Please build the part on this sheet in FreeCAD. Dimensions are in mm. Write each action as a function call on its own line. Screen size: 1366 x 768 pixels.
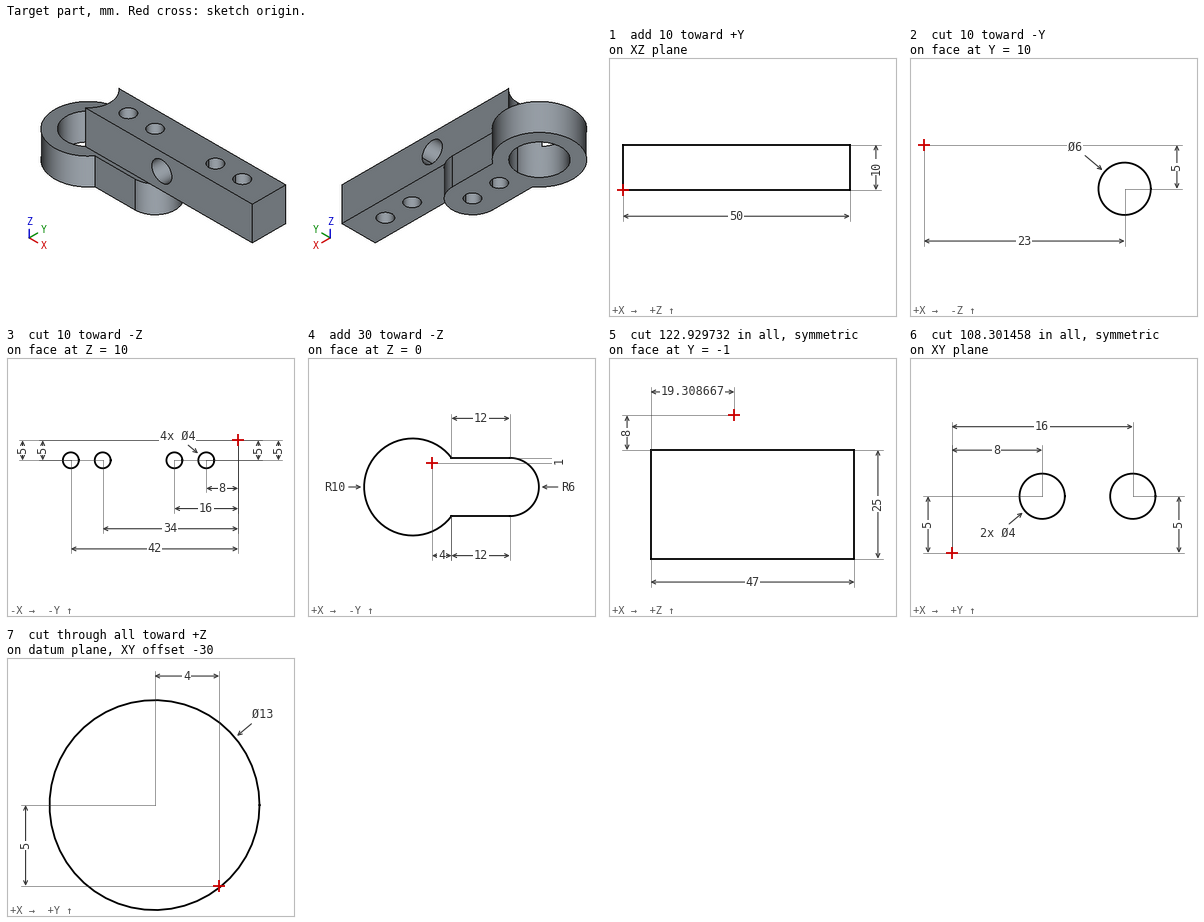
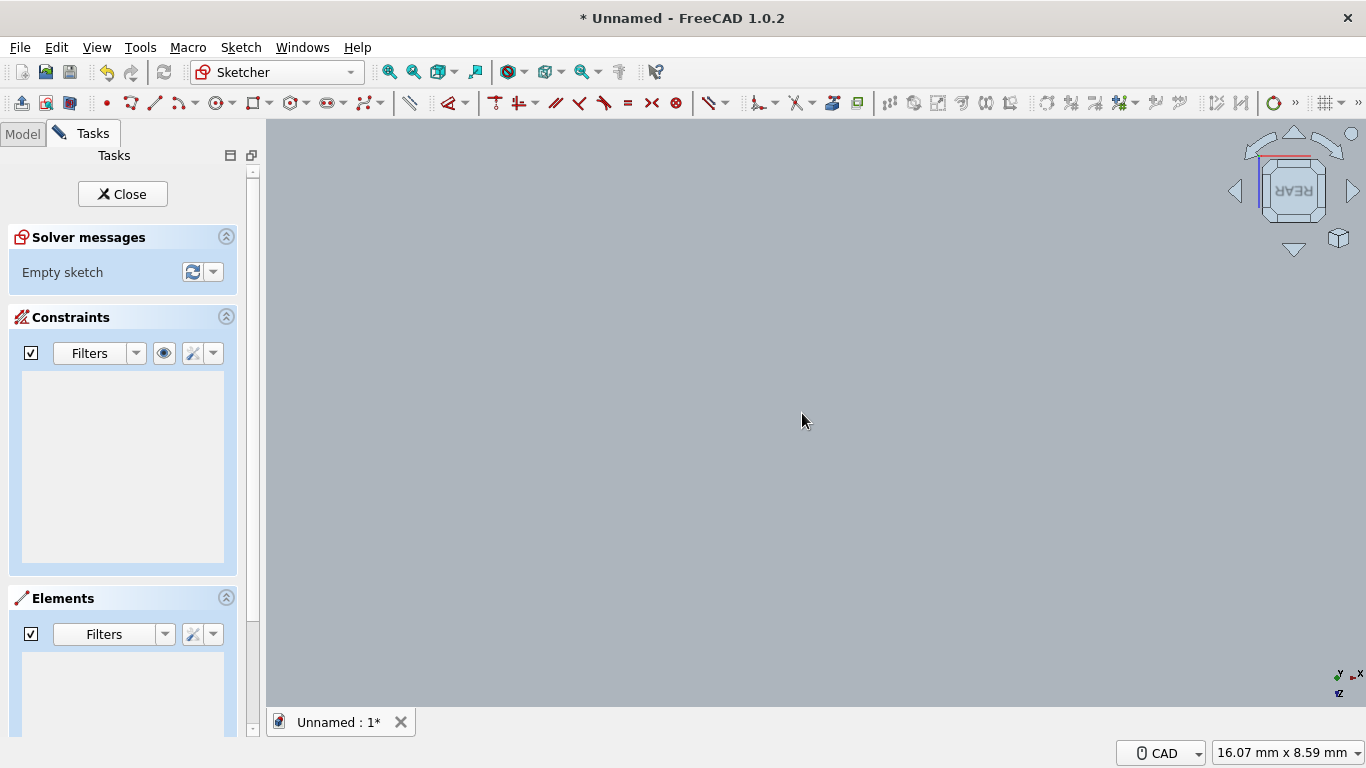
click(216, 104)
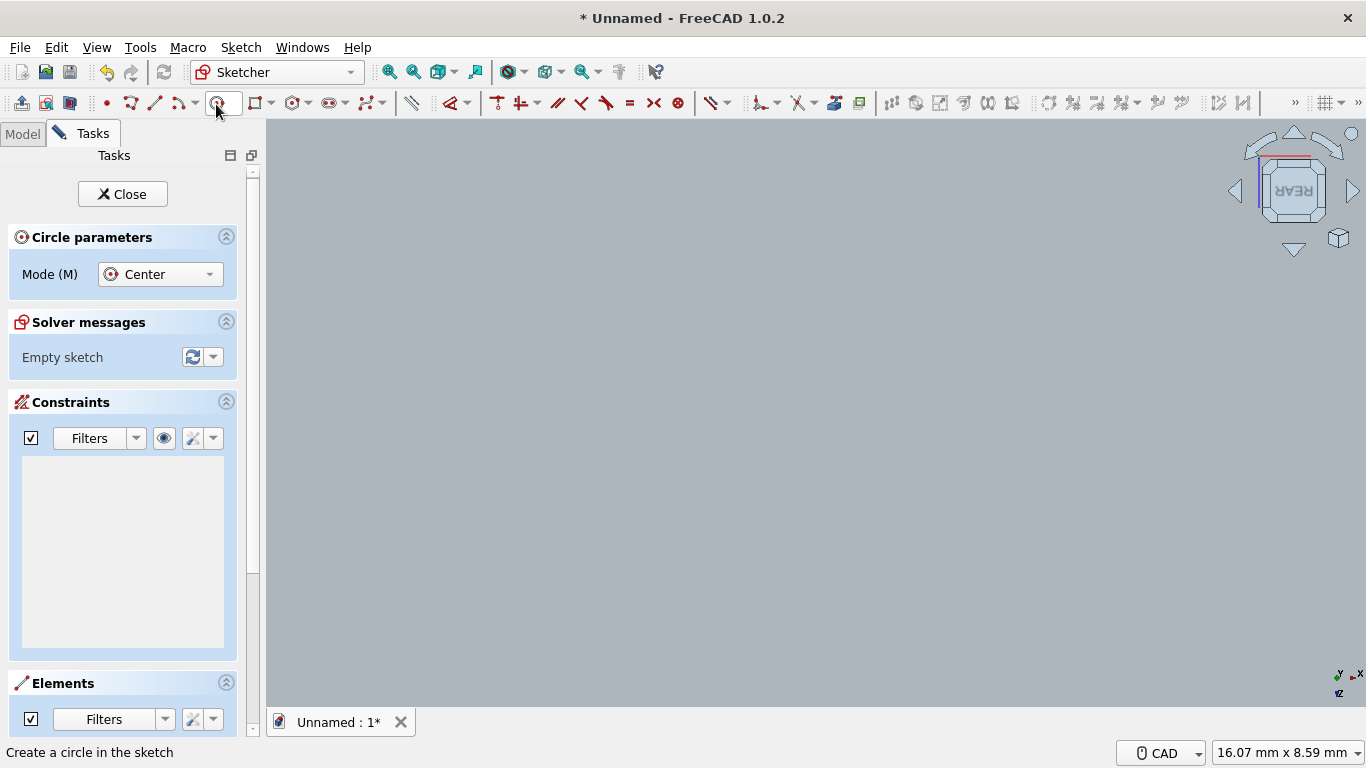
click(747, 410)
move(893, 265)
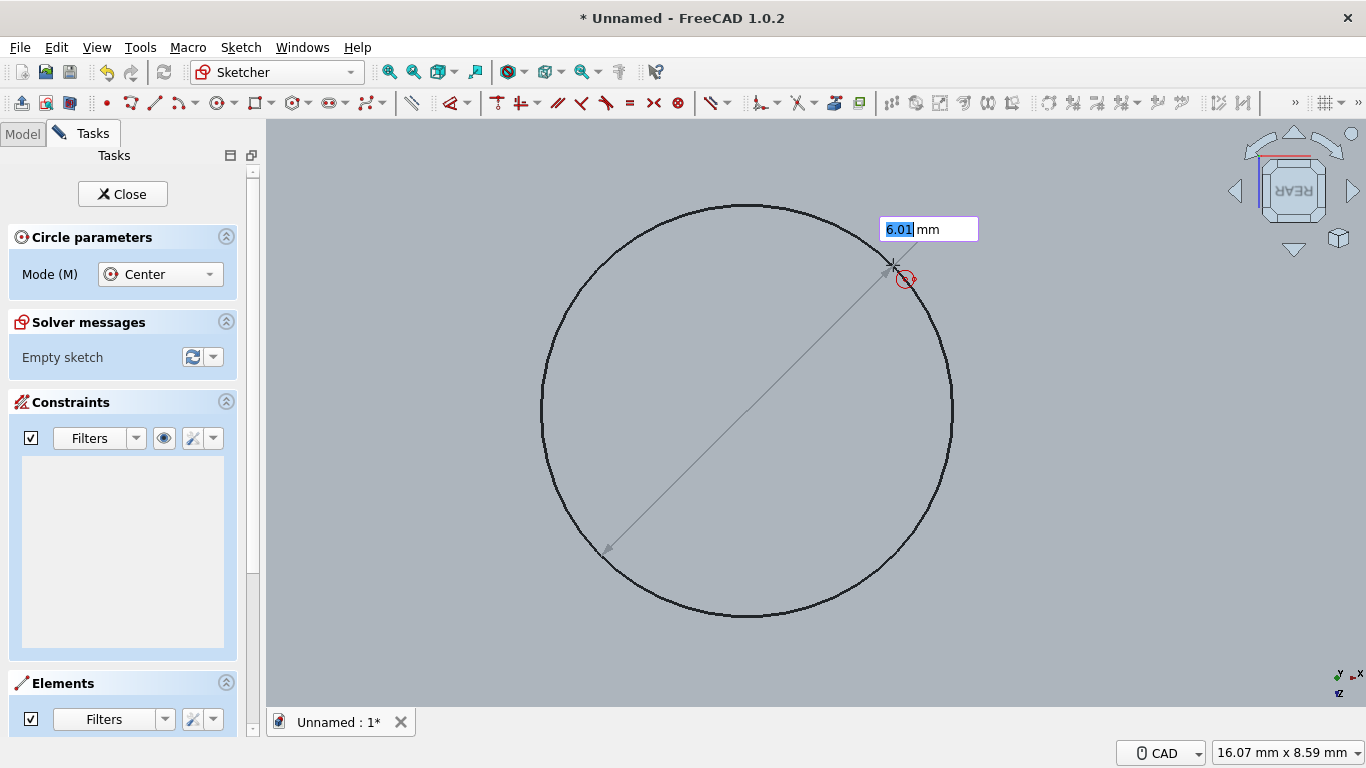
text(6)
key(Return)
key(Escape)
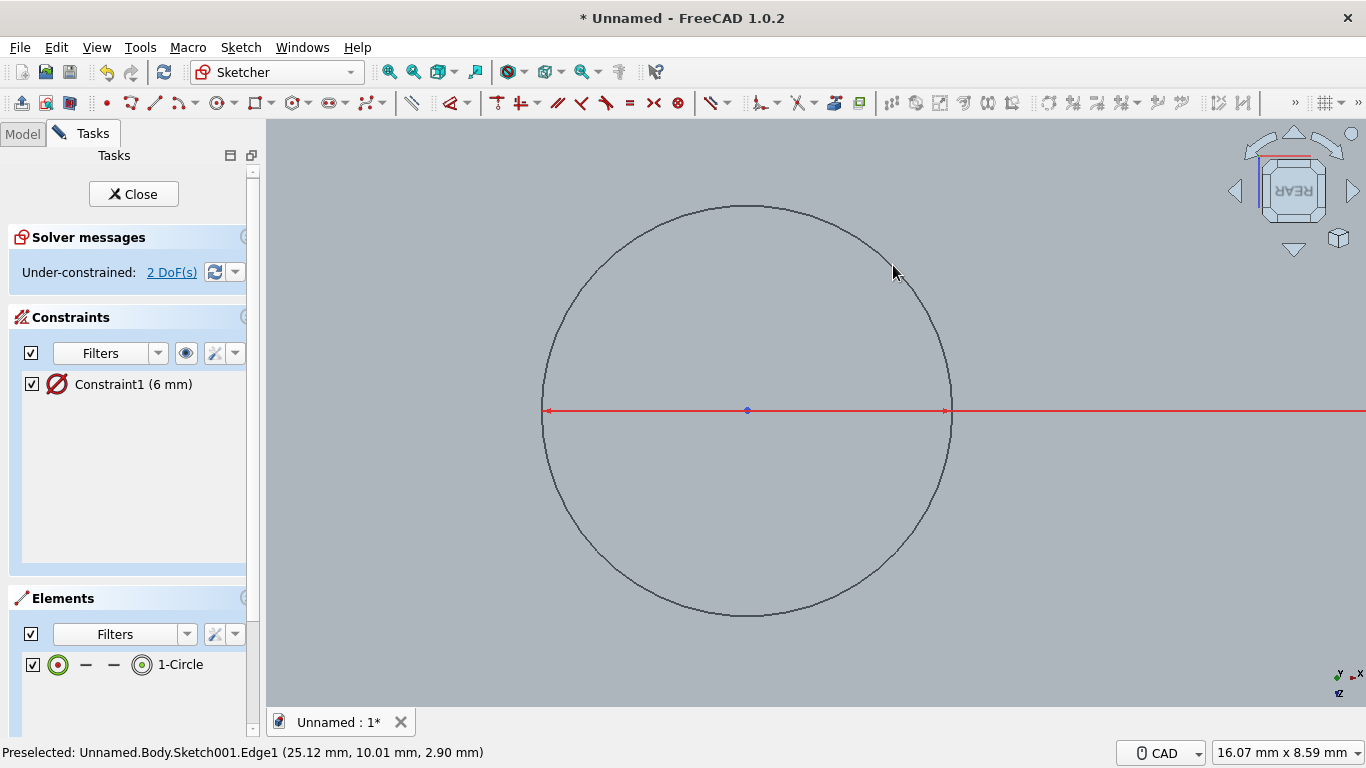
click(450, 104)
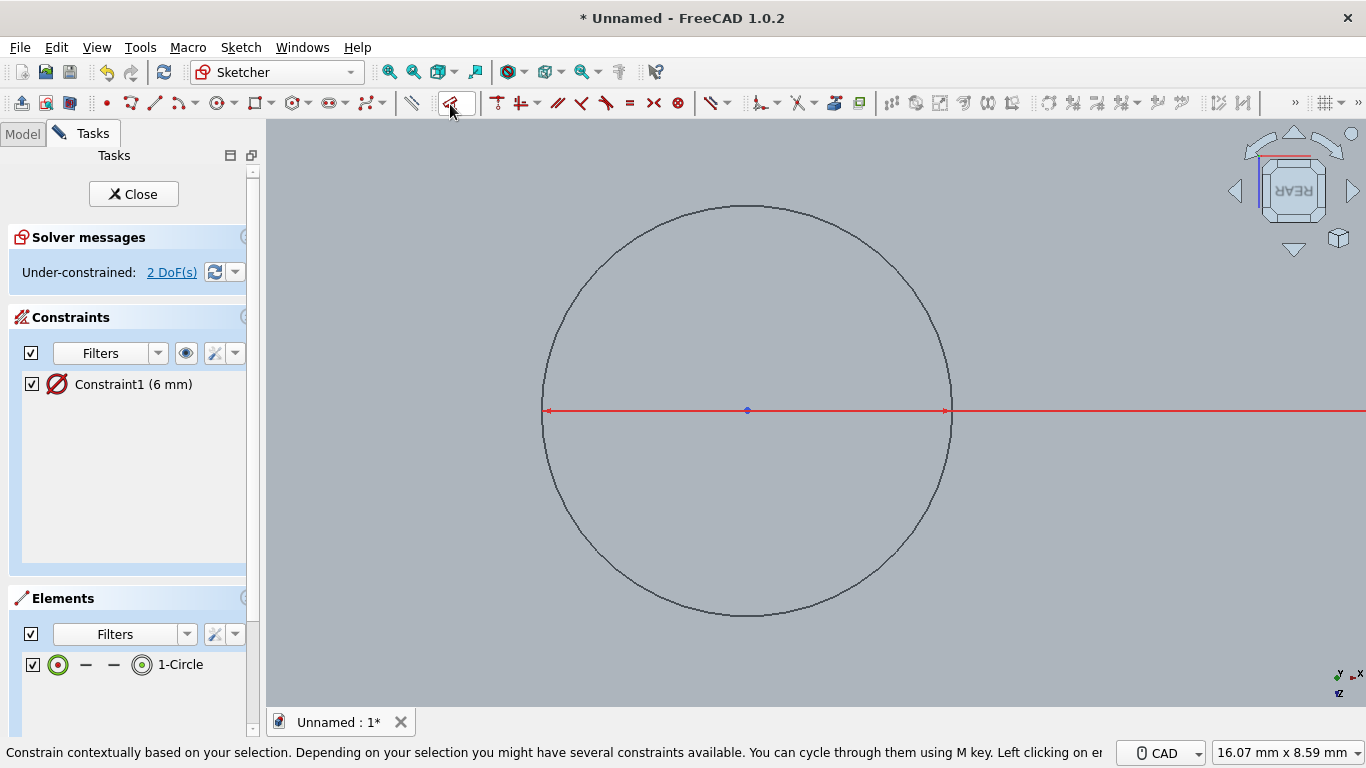
click(747, 411)
click(781, 279)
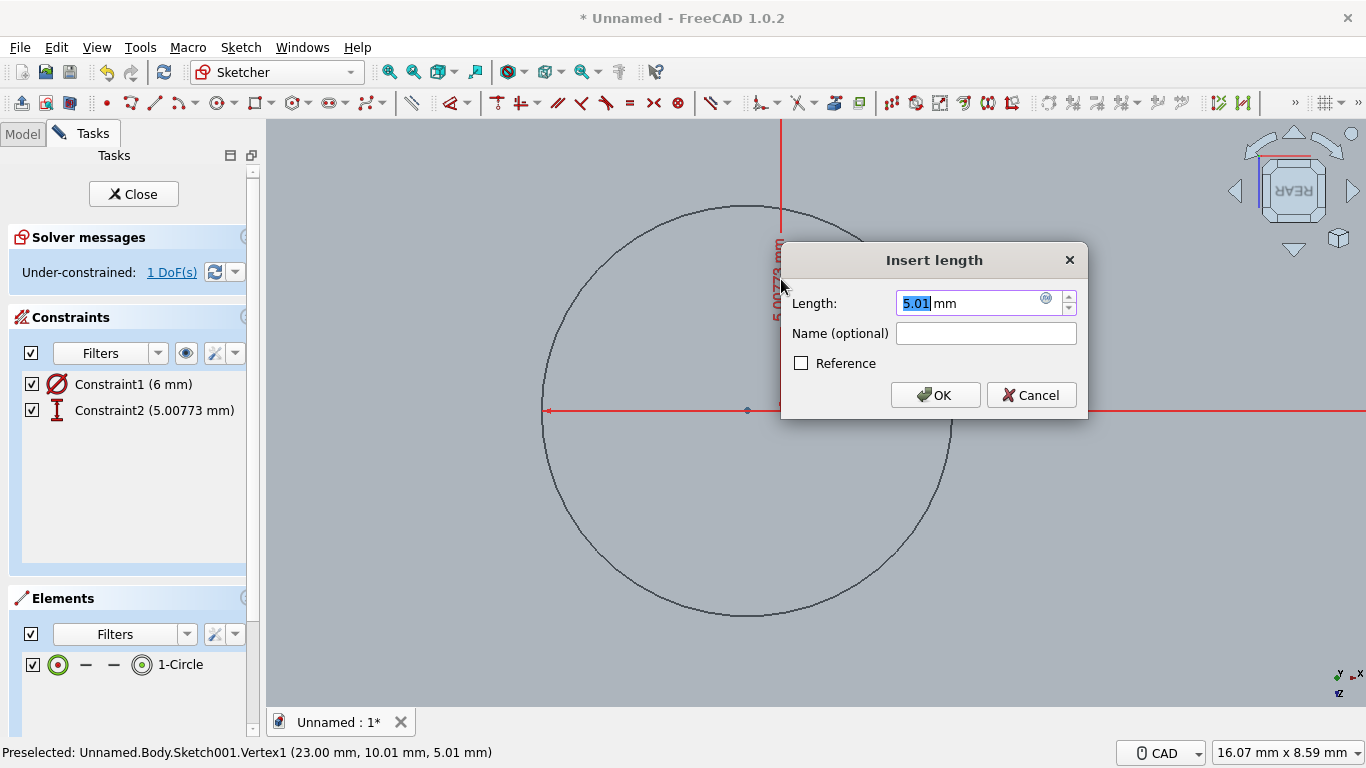
text(5)
key(Return)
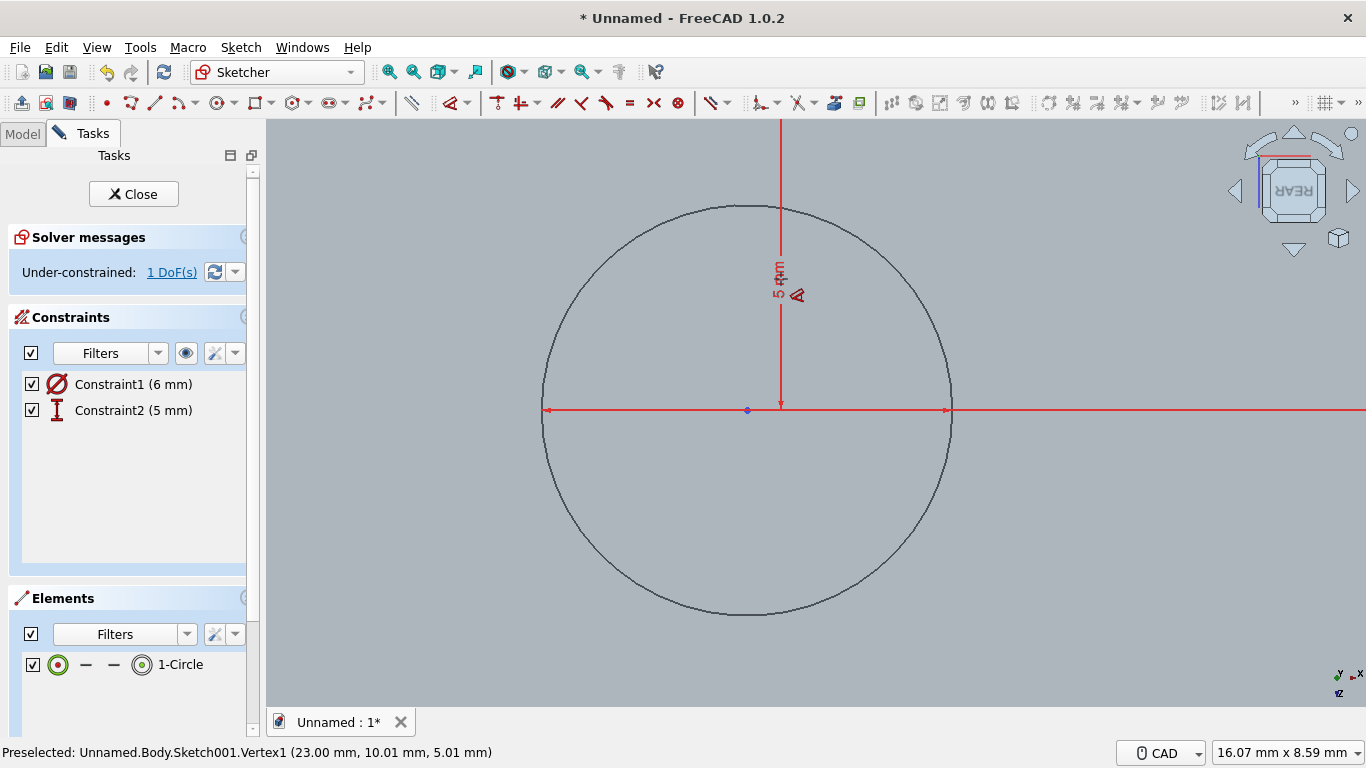
click(747, 410)
click(521, 444)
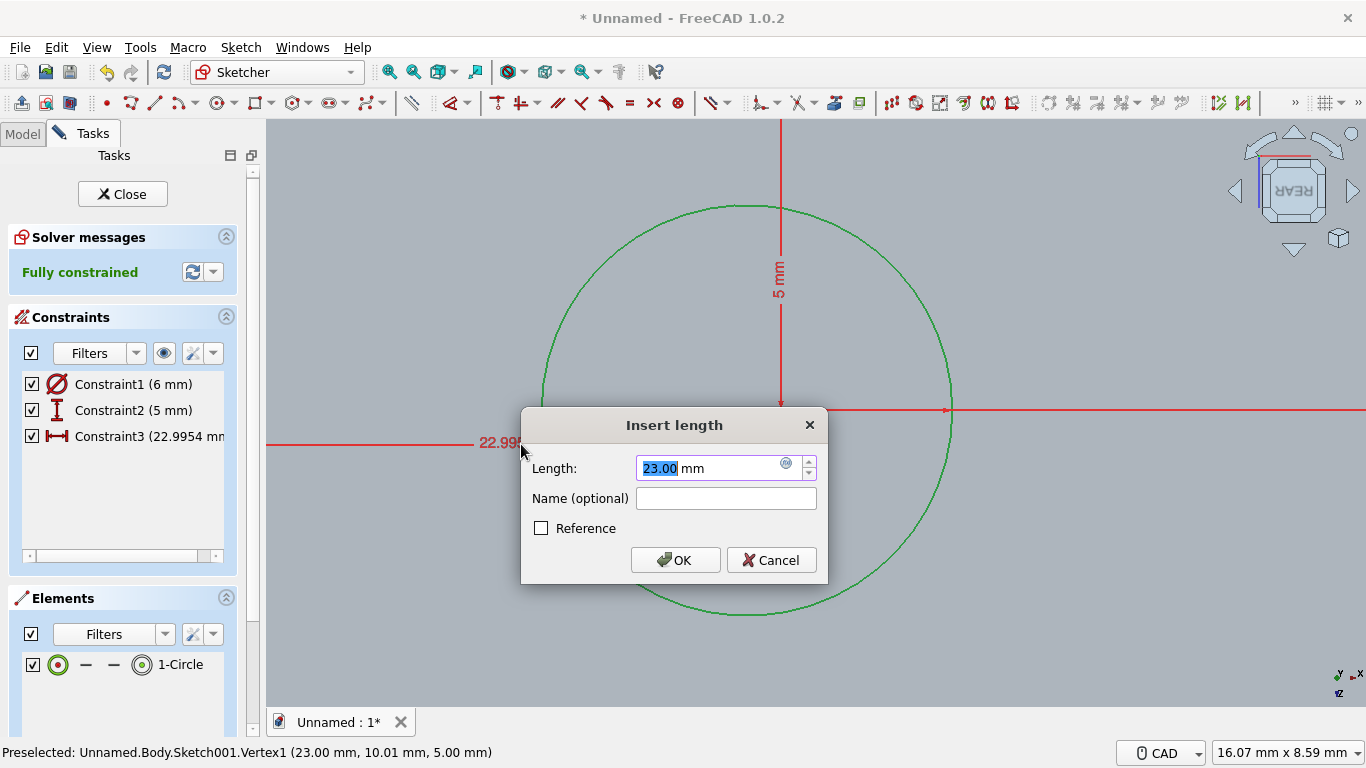
text(23)
key(Return)
key(Escape)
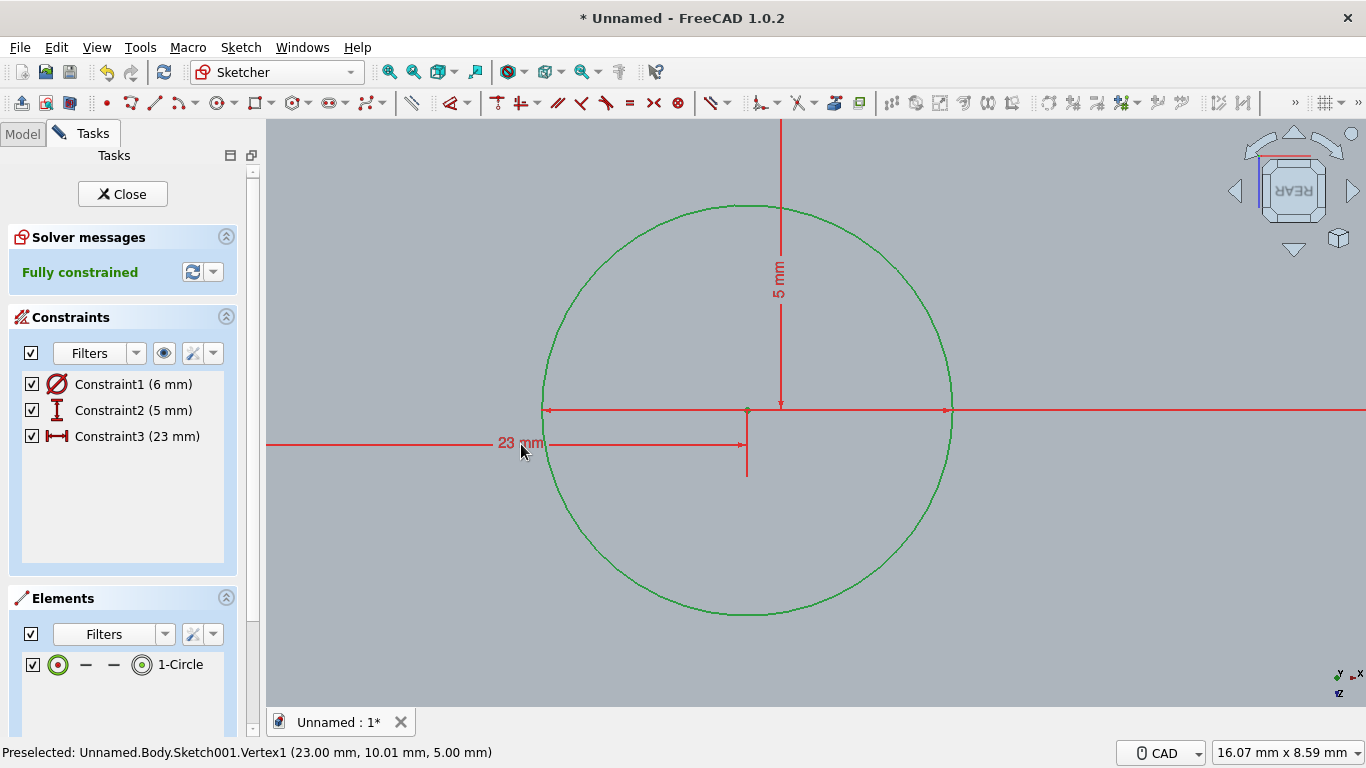
click(123, 194)